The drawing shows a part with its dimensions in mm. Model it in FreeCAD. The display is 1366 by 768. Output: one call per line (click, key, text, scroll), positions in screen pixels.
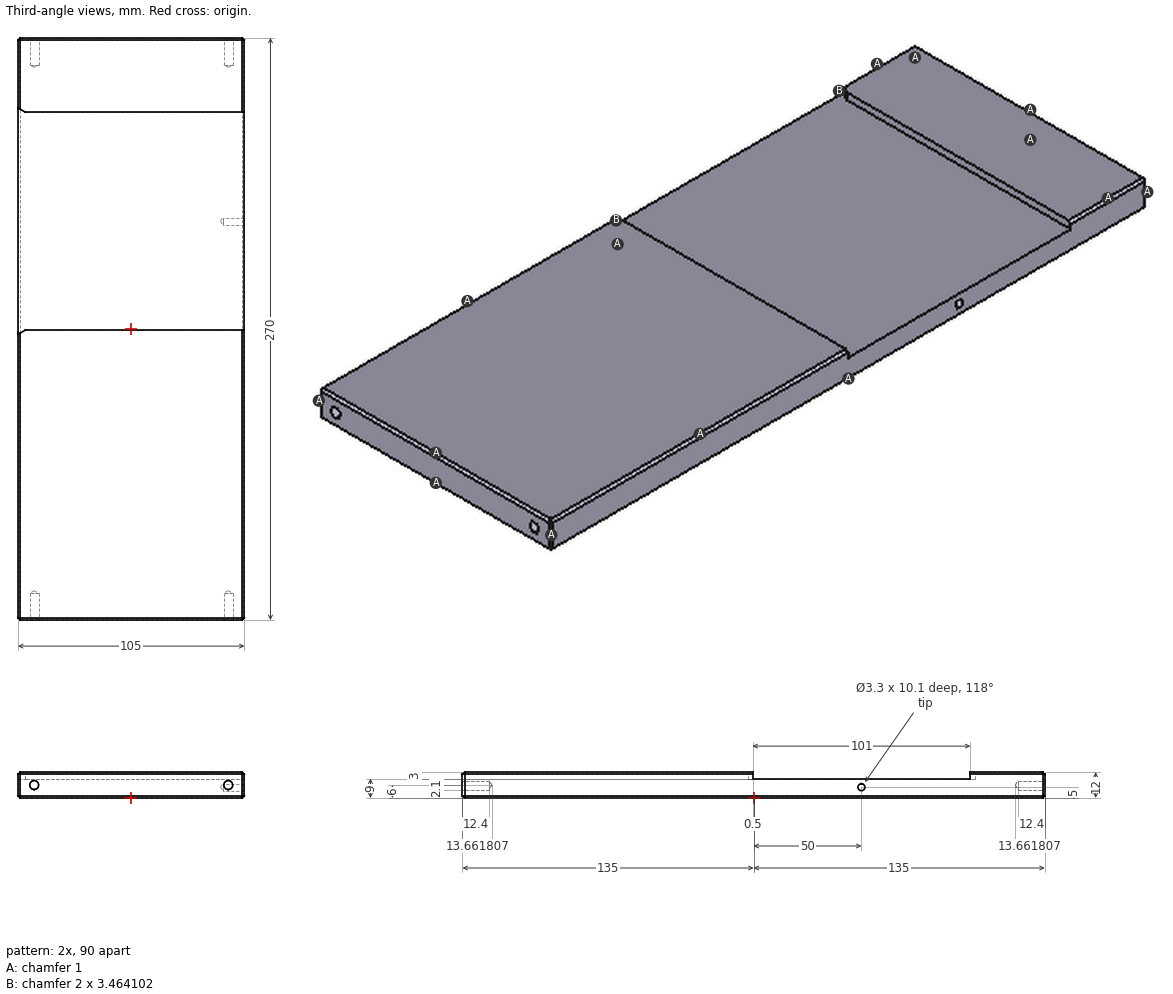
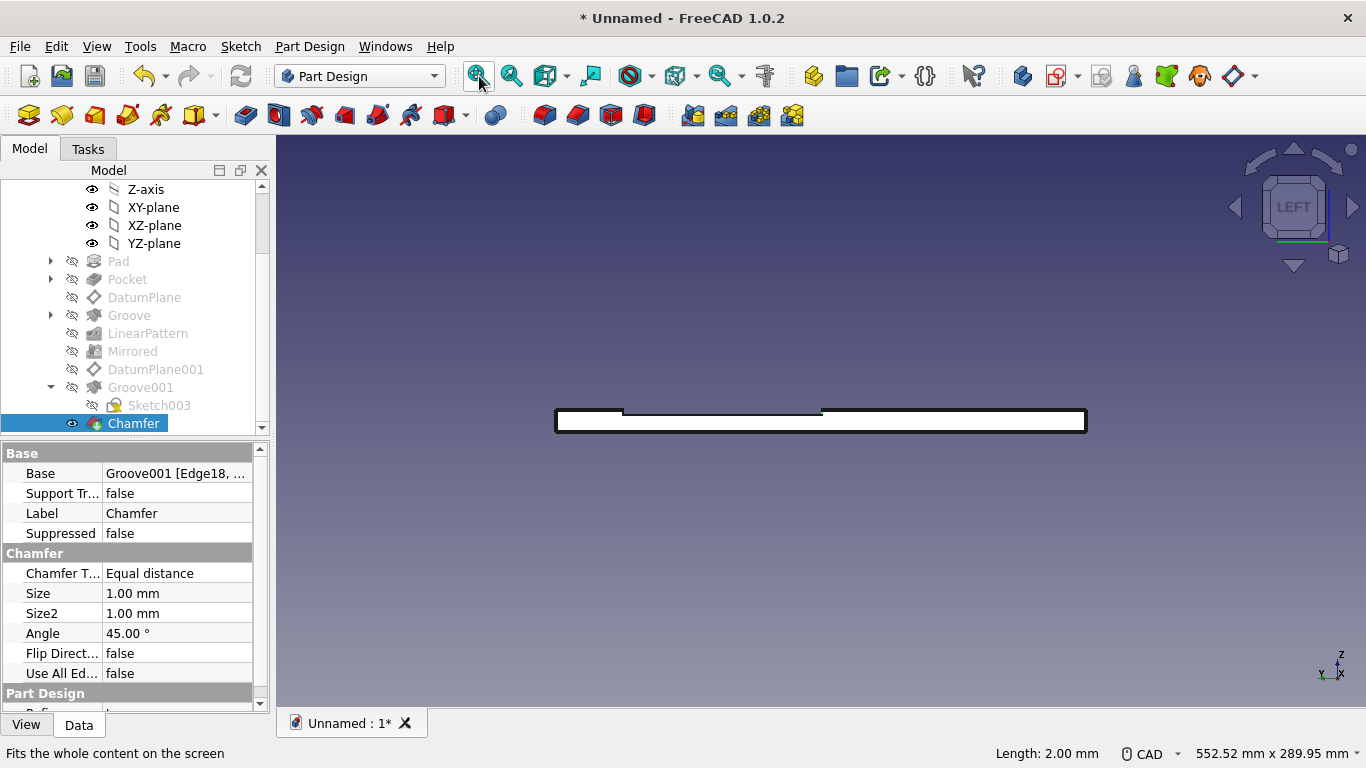
key(v)
key(3)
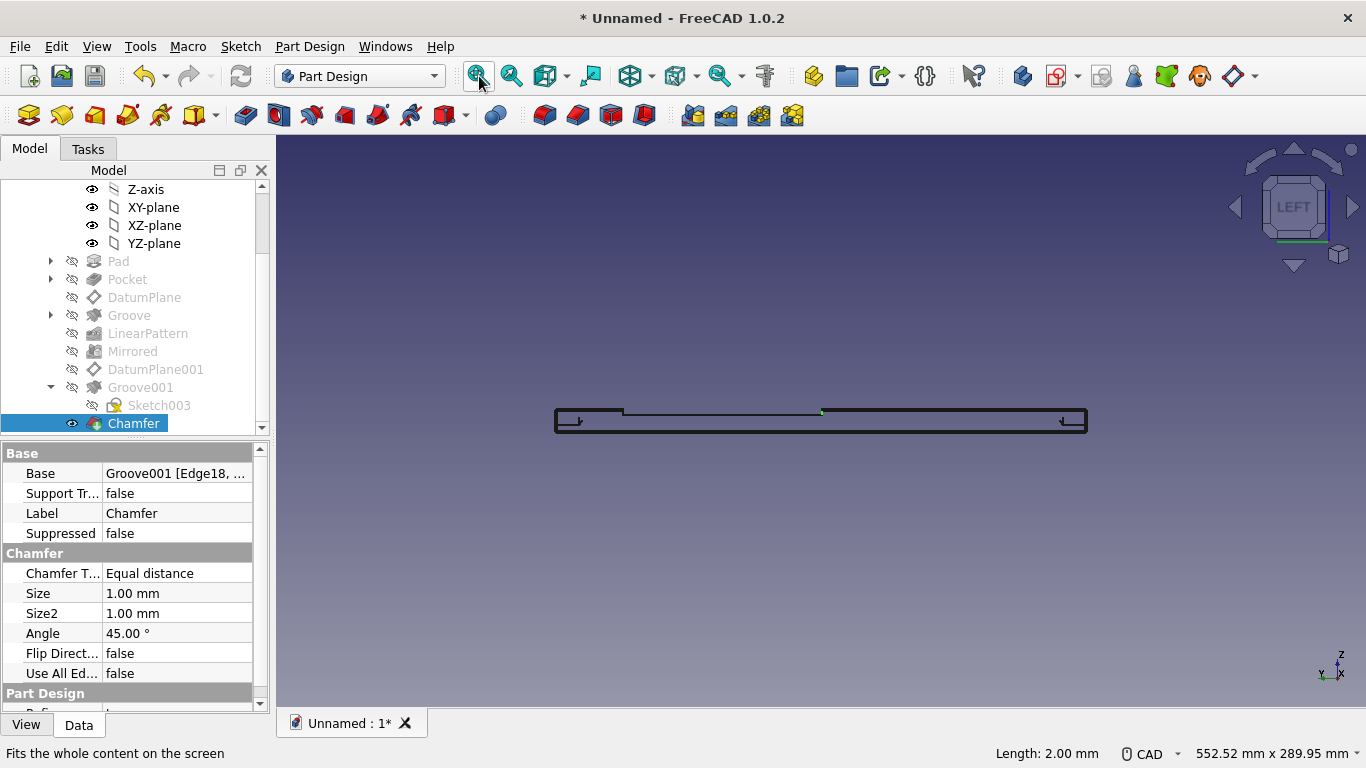
key(0)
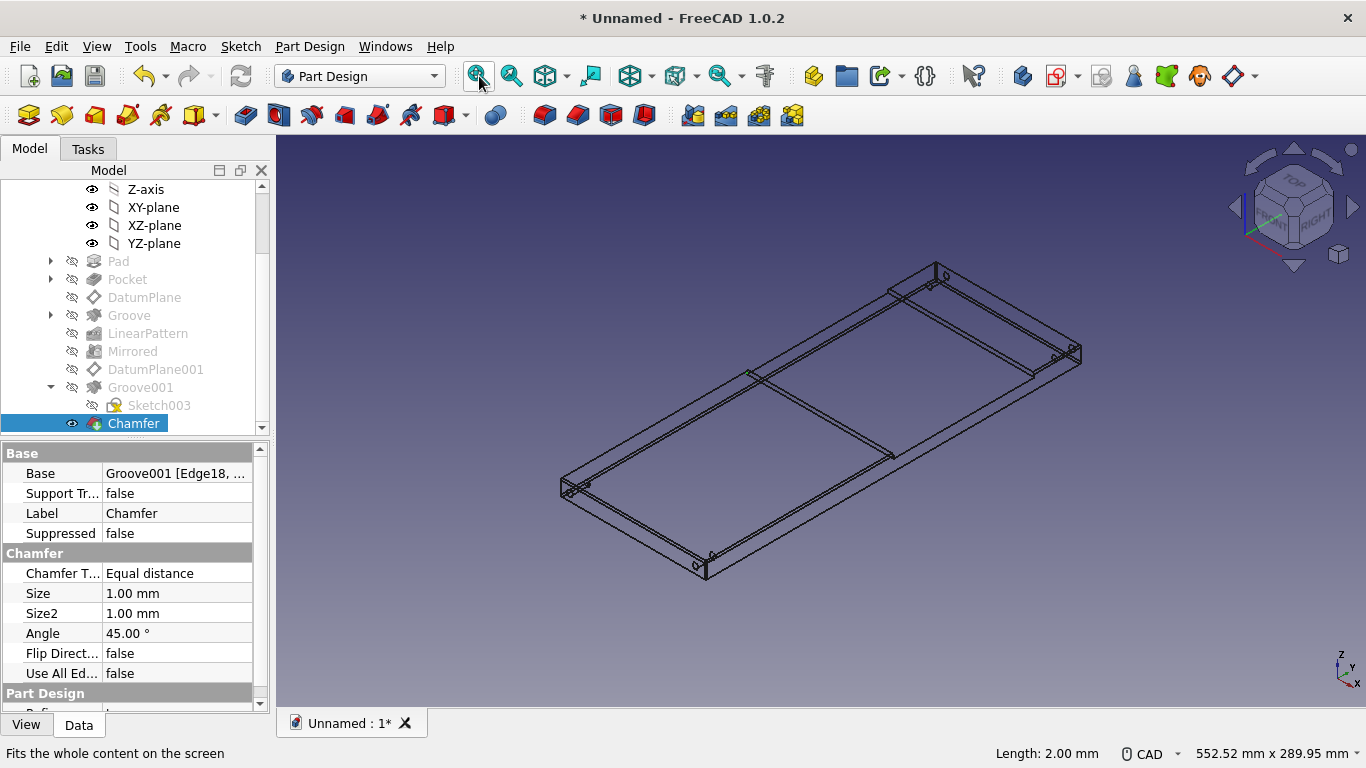
scroll(888, 290, up, 12)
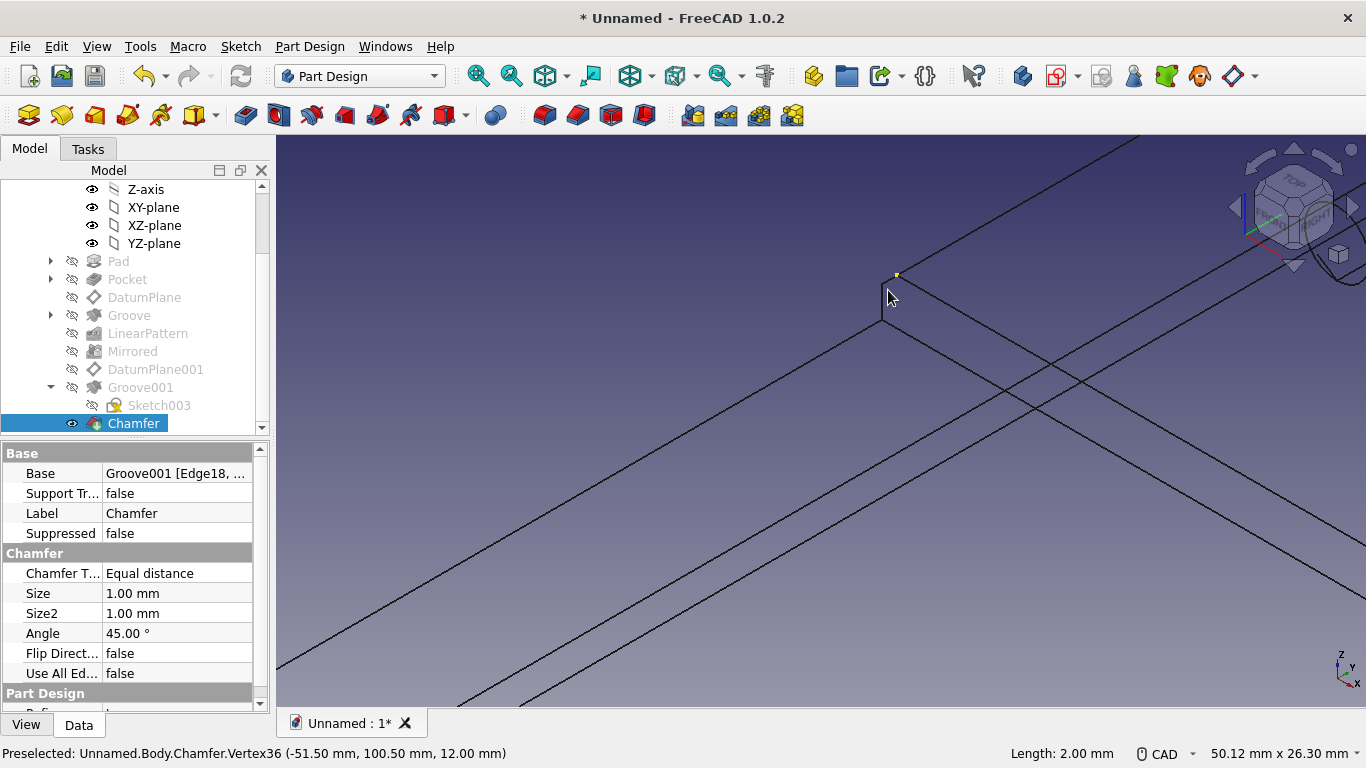
click(882, 301, ctrl)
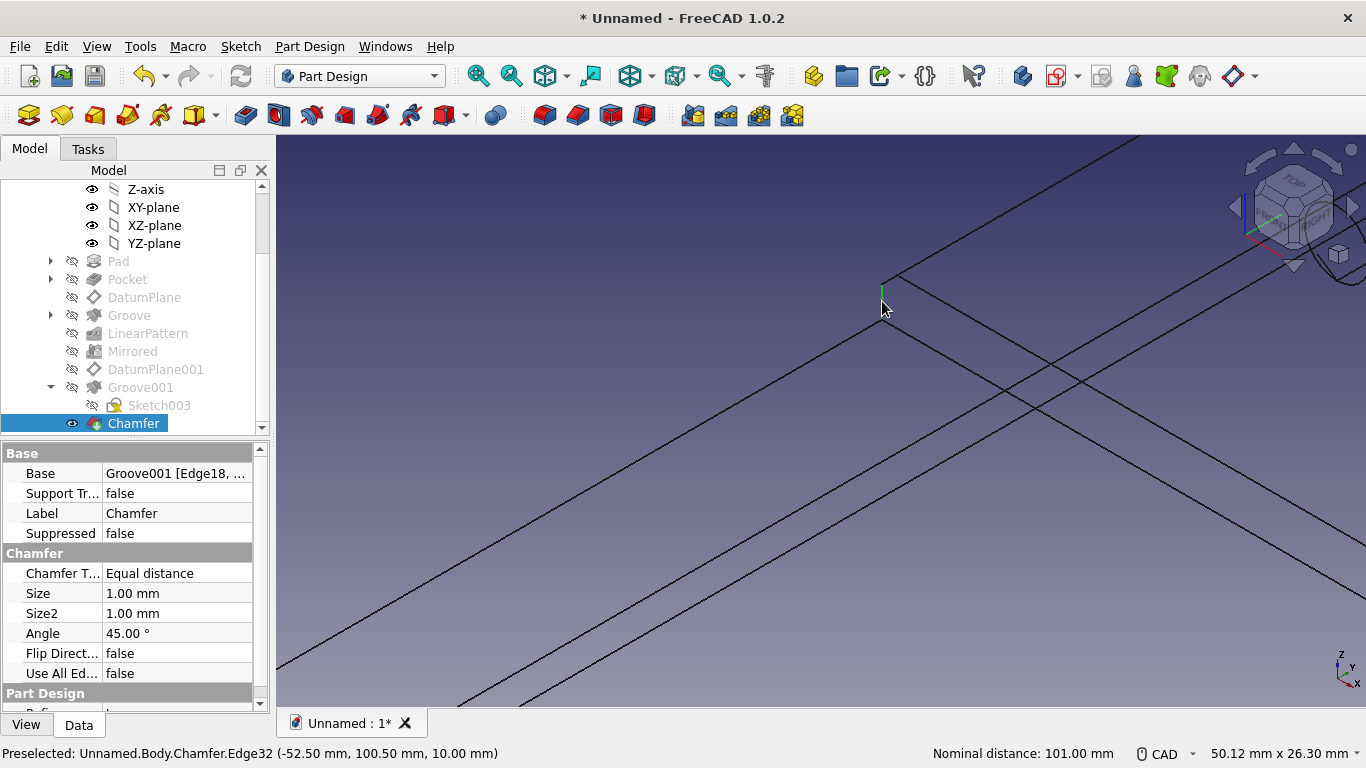
key(v)
key(1)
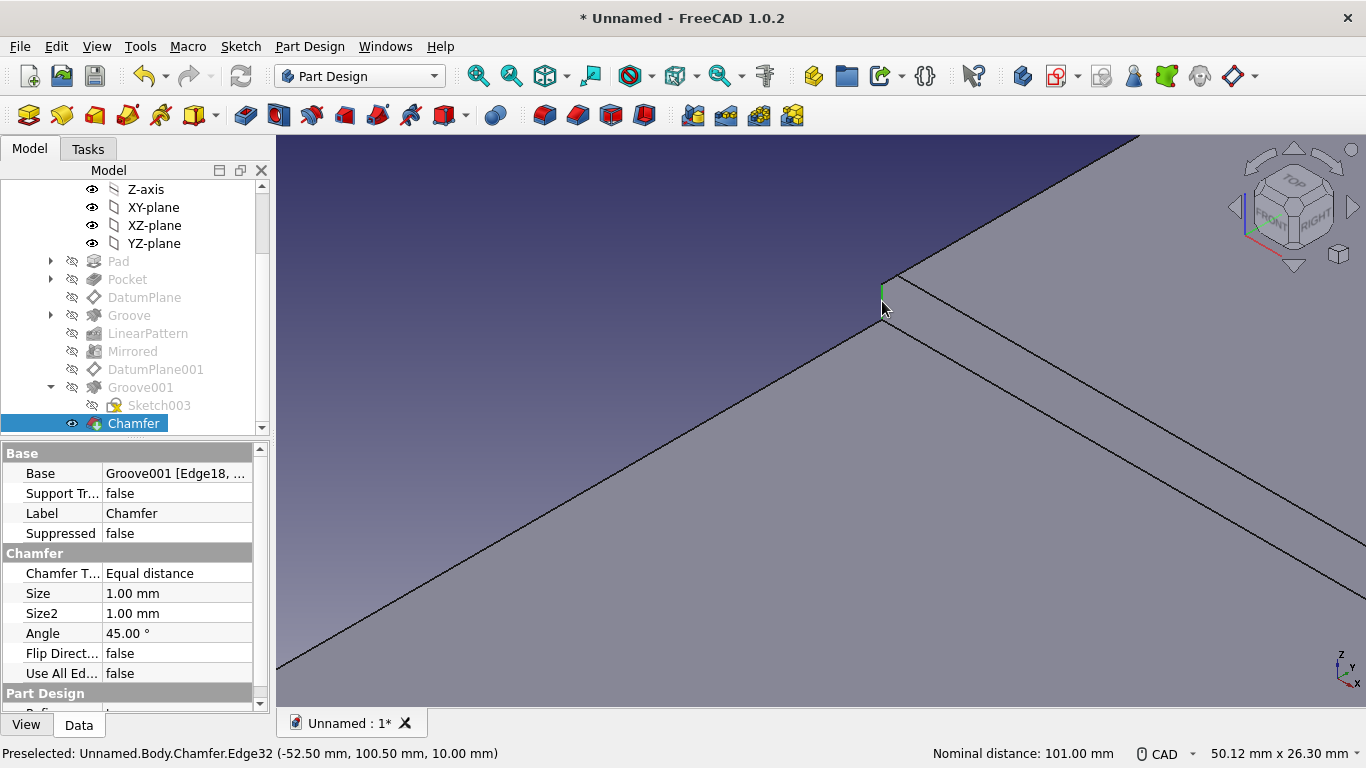
click(578, 116)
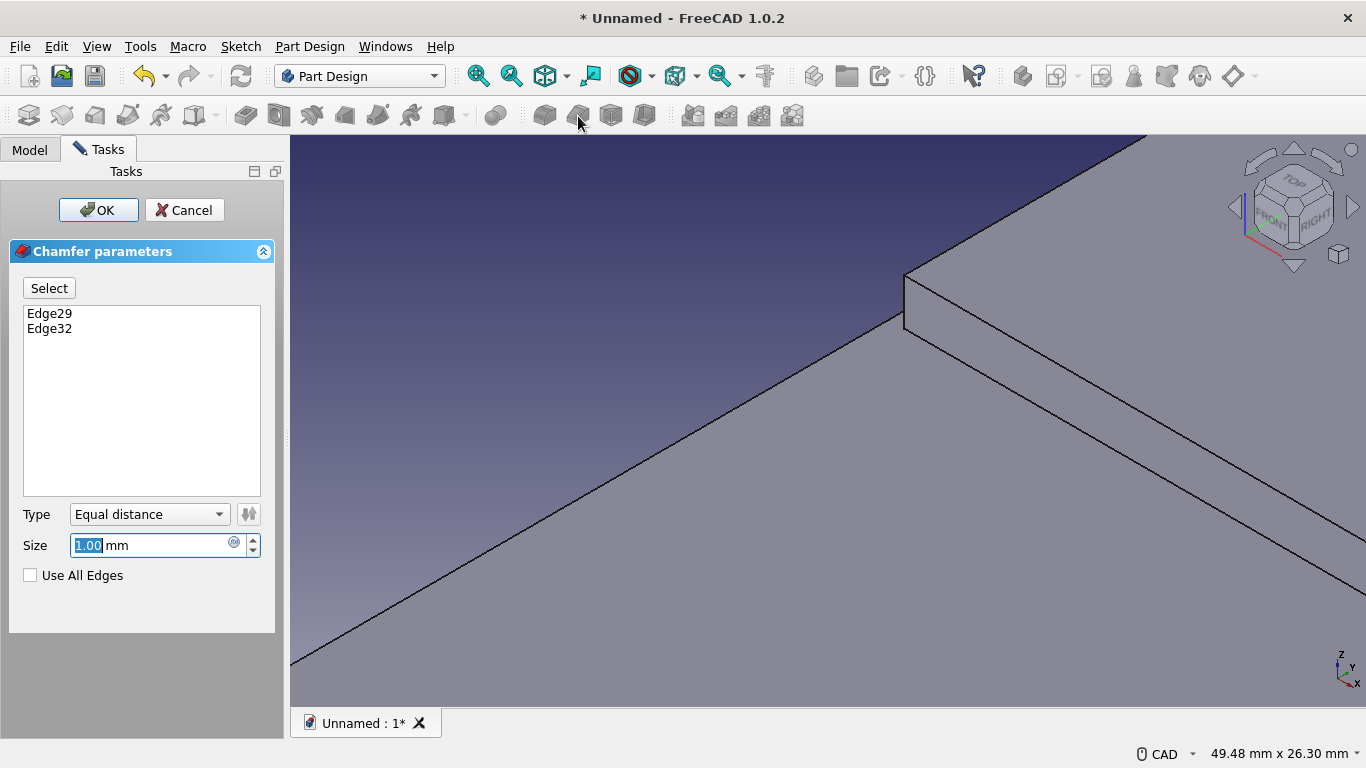
text(2)
key(Tab)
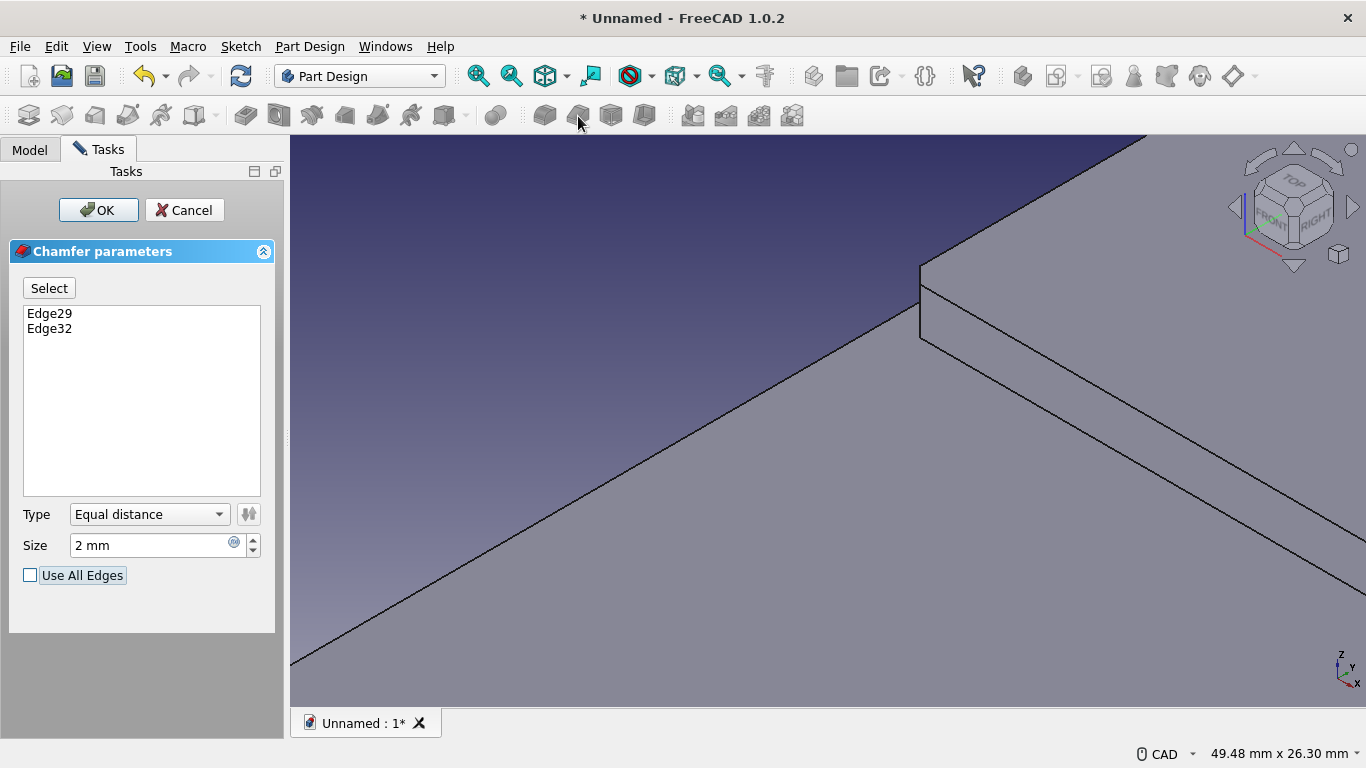
click(150, 514)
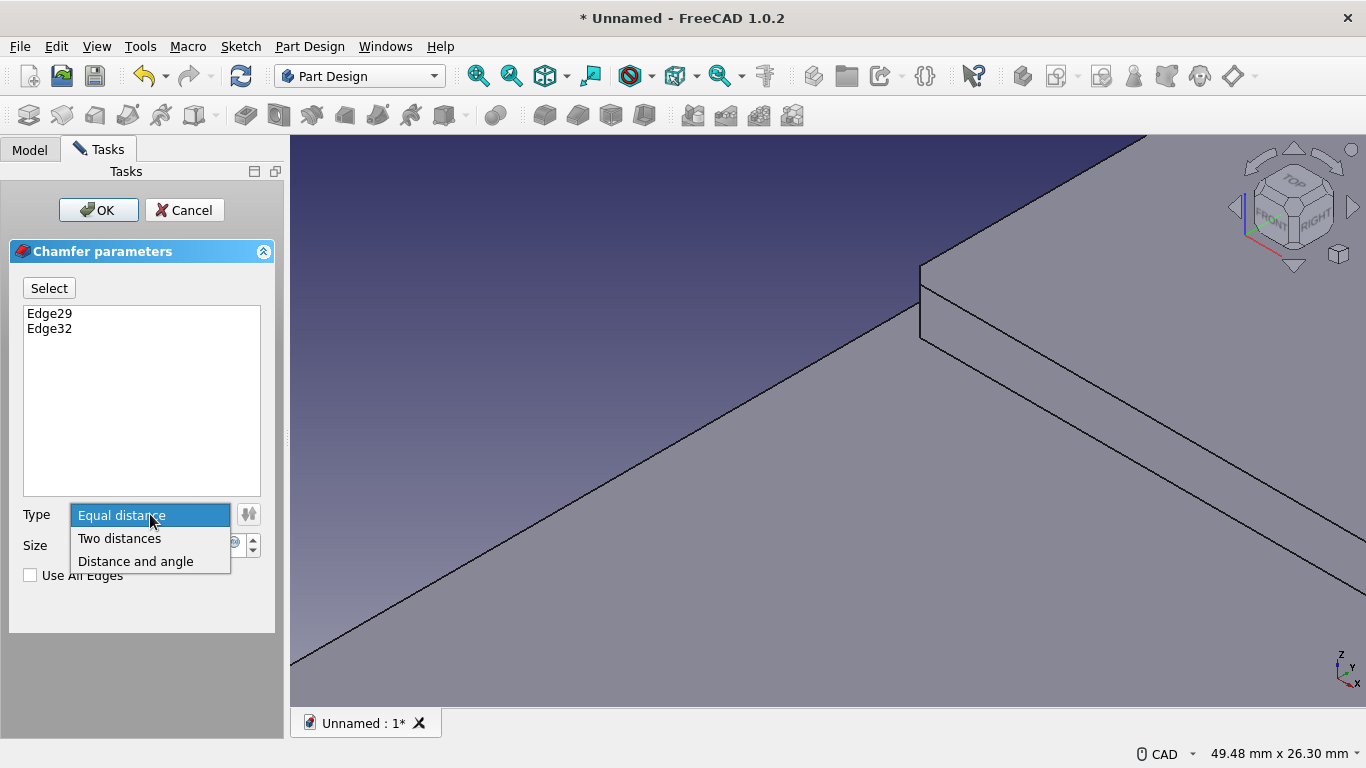
click(148, 538)